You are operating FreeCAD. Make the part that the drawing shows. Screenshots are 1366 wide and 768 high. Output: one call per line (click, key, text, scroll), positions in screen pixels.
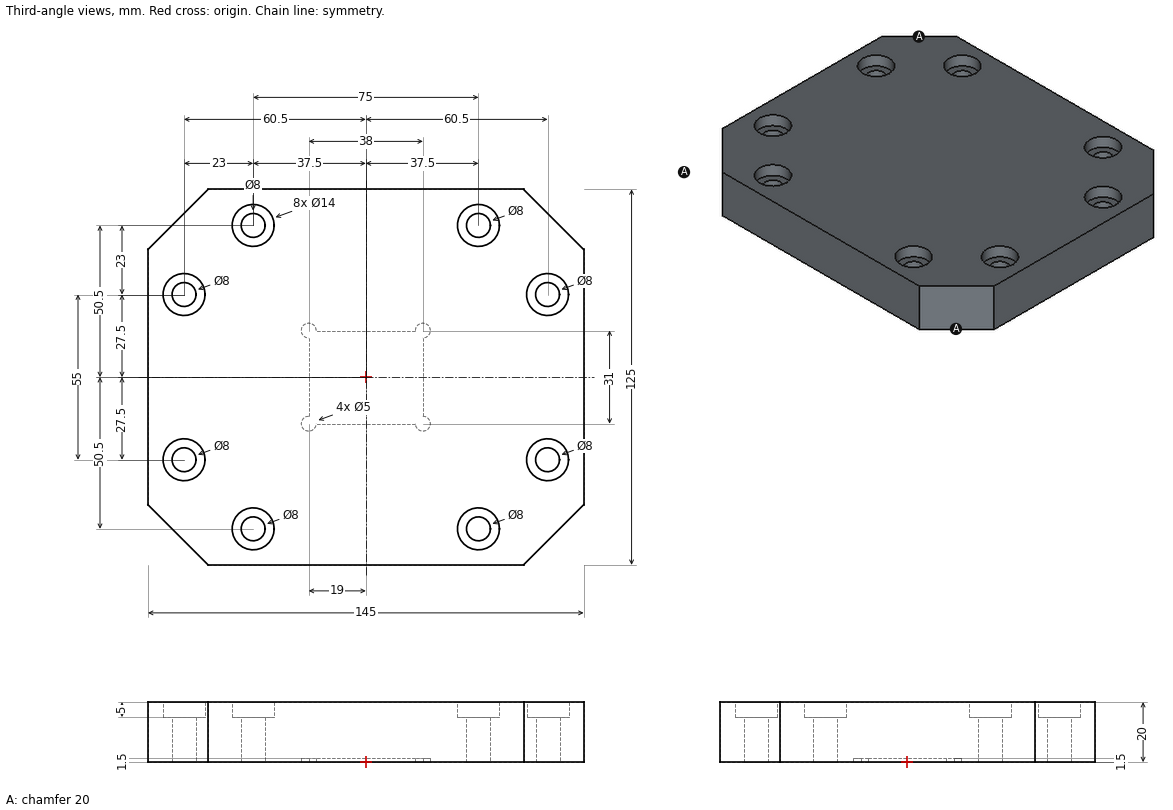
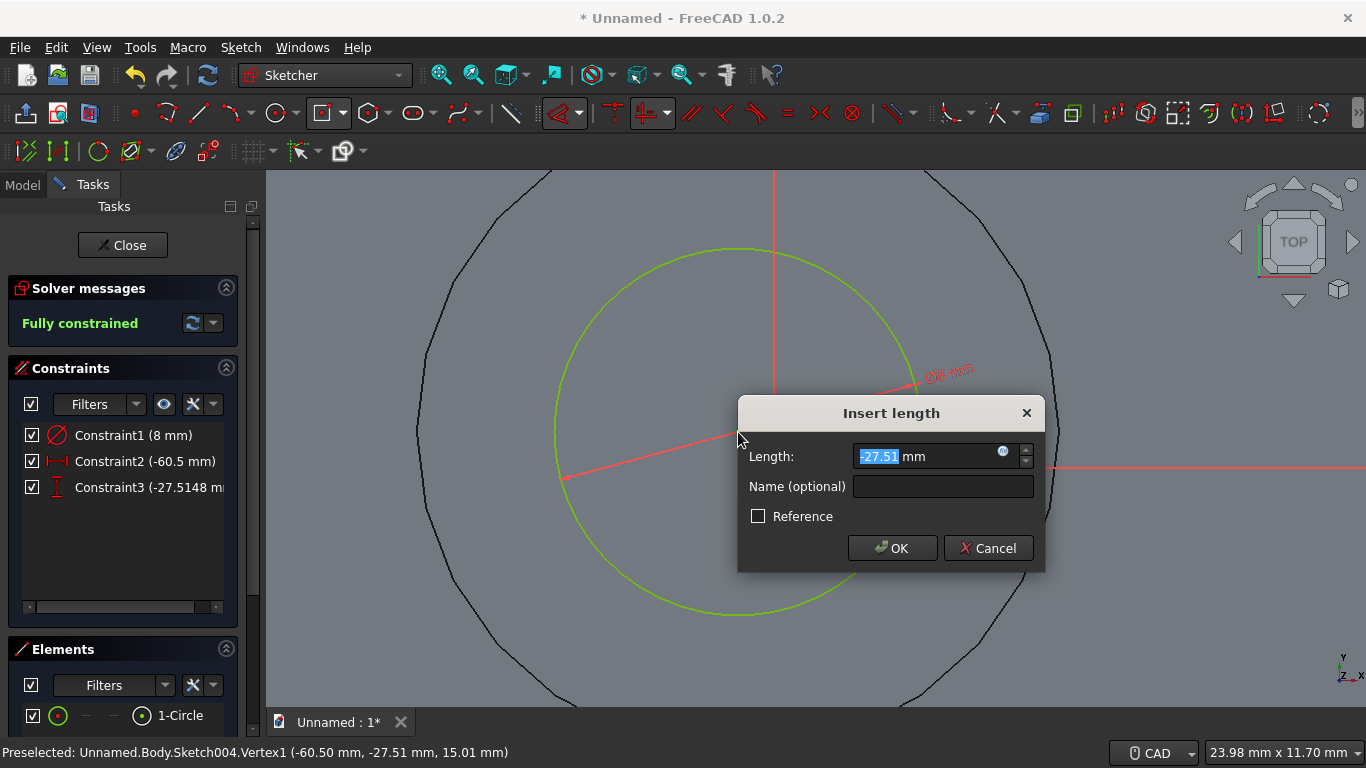
text(-27.5)
key(Return)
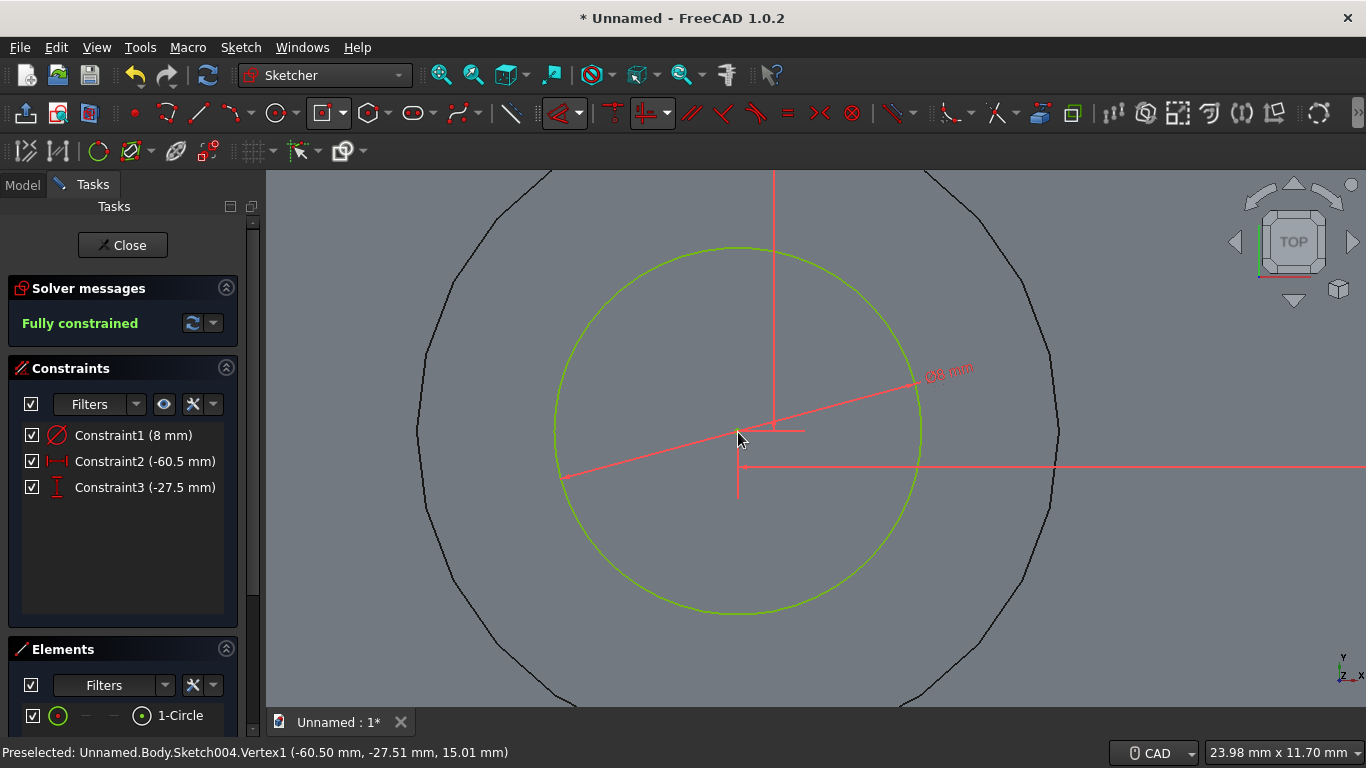
click(123, 245)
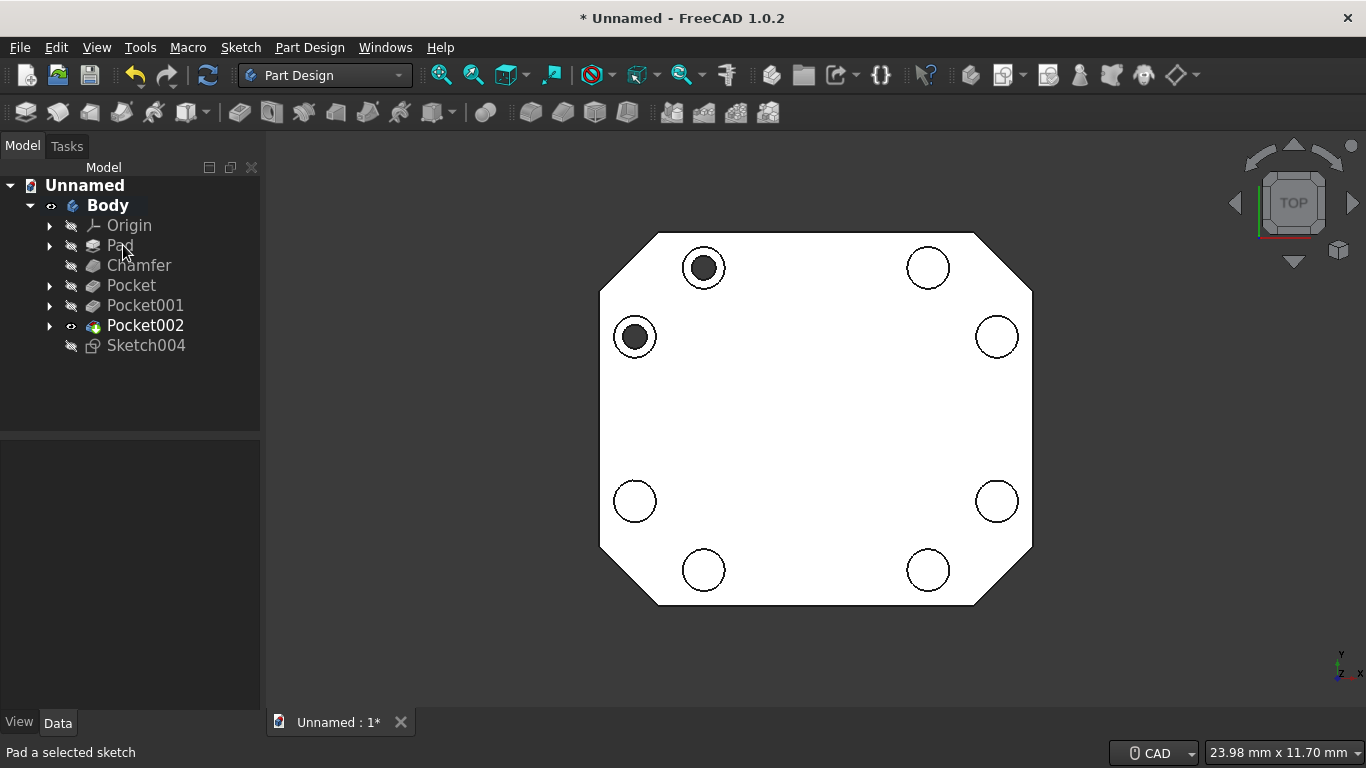
click(240, 112)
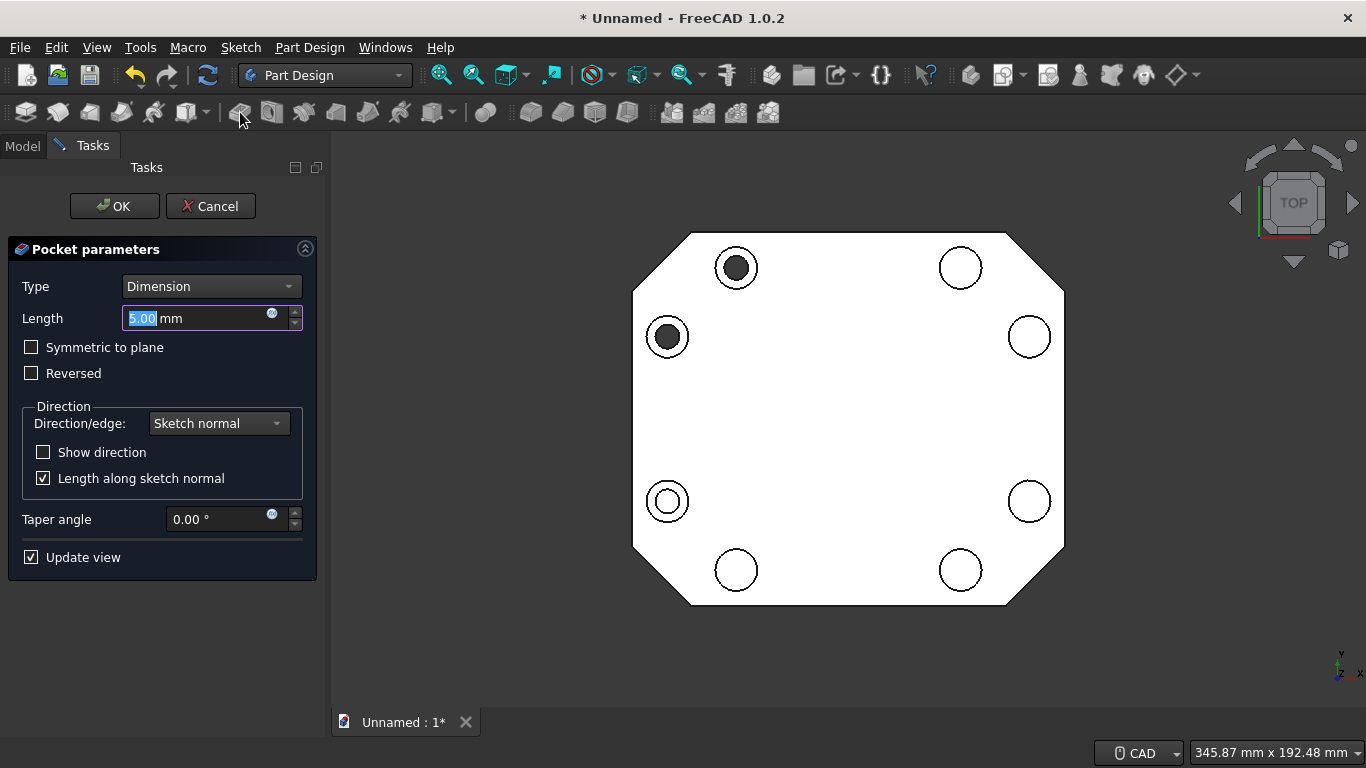
click(212, 286)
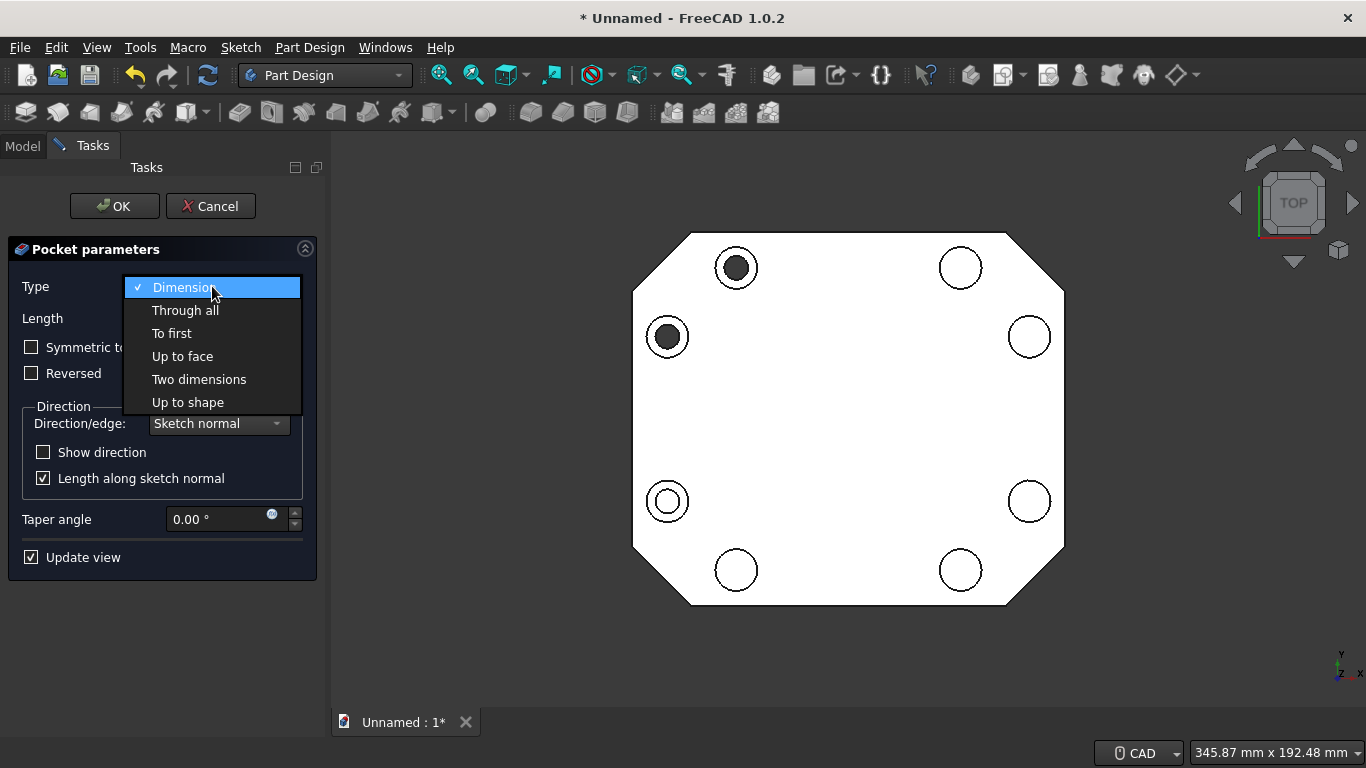
click(212, 334)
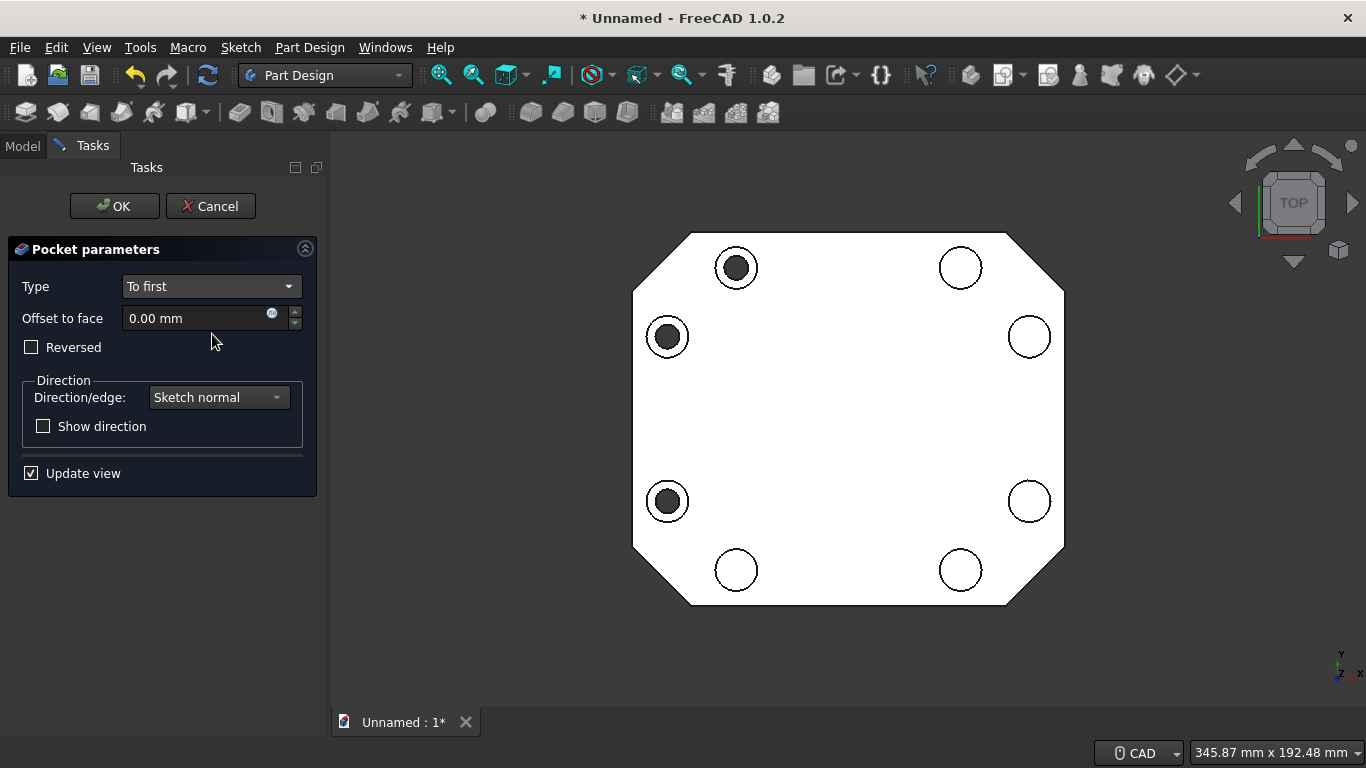
click(115, 206)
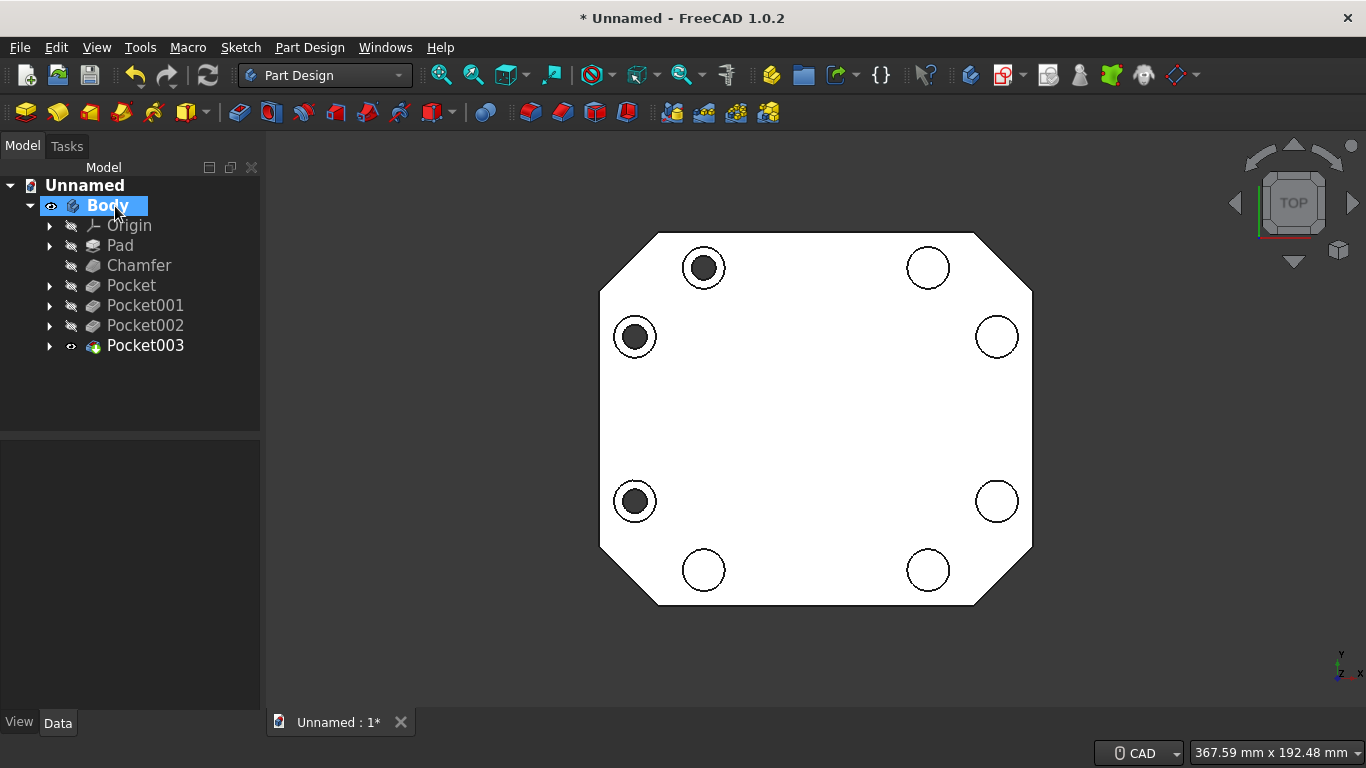
click(928, 267)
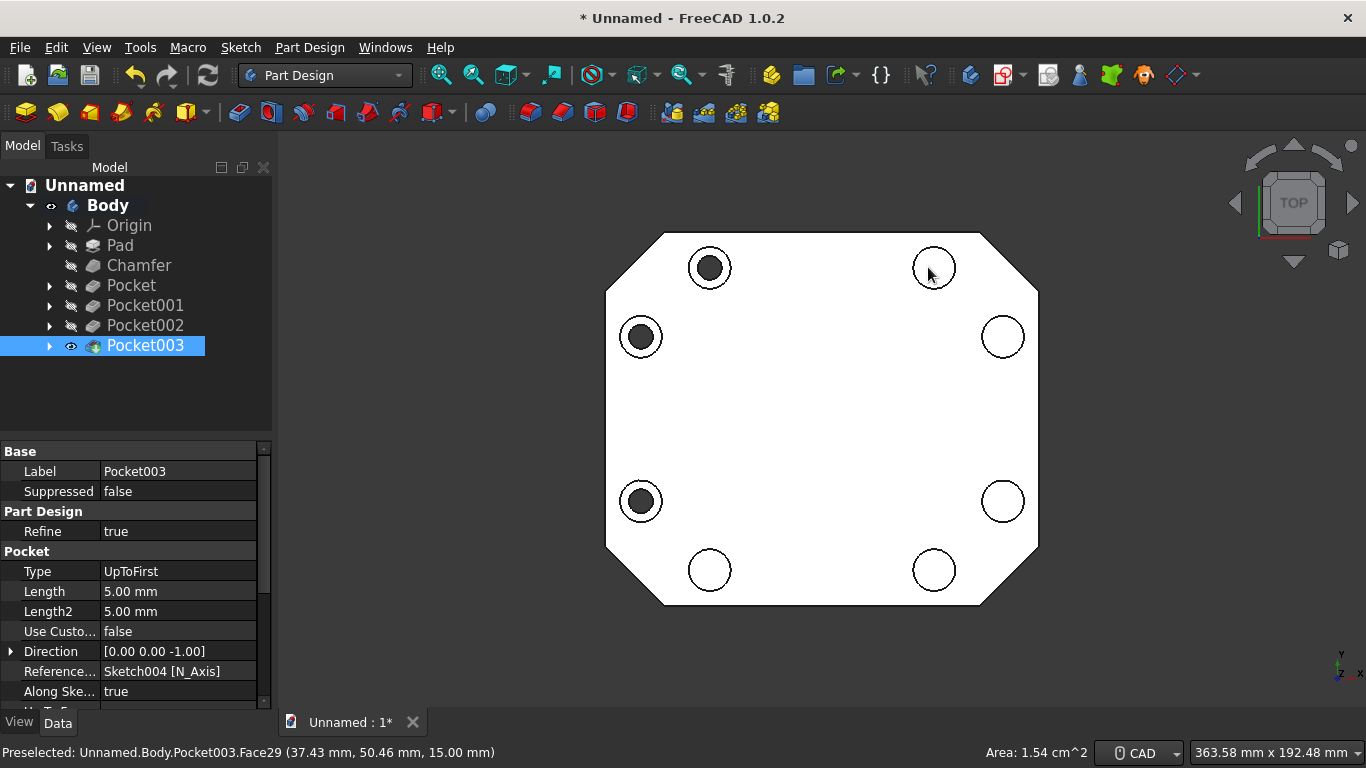
click(1004, 76)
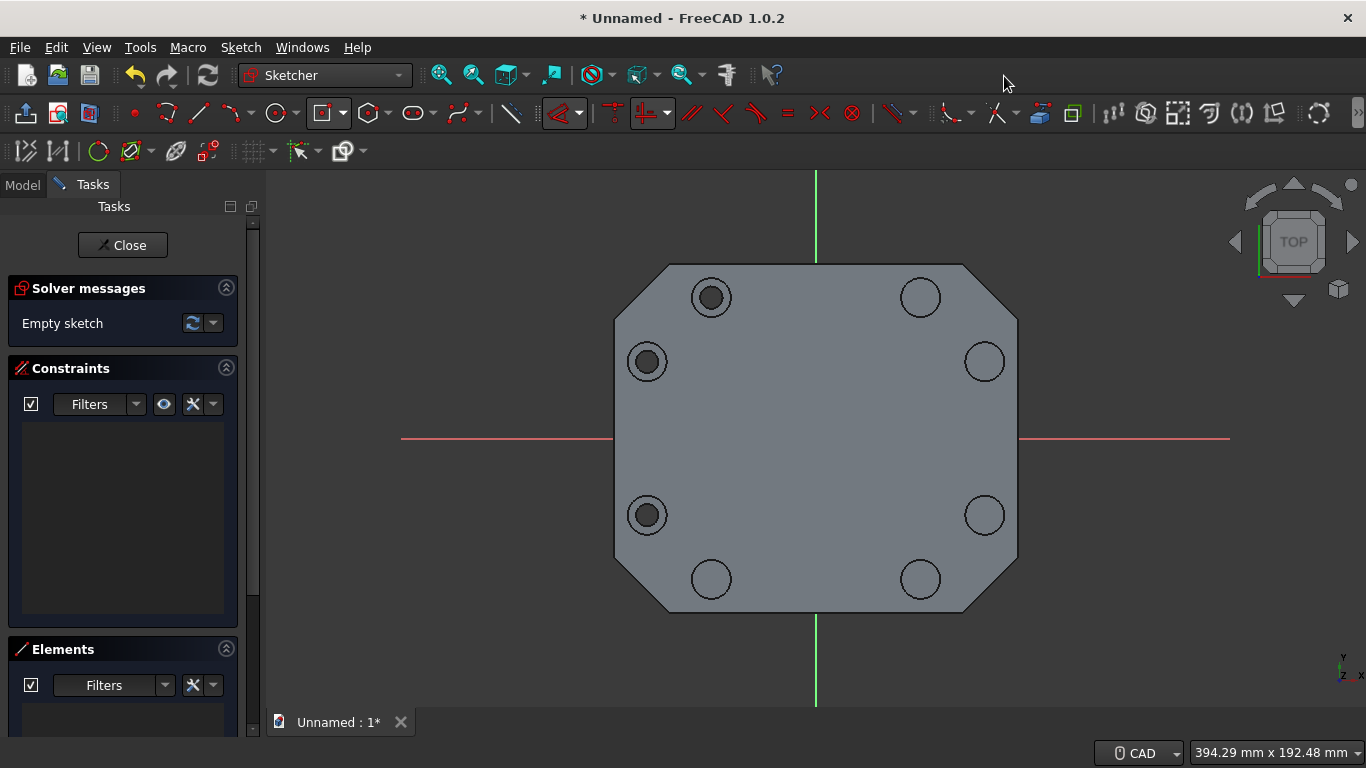
scroll(709, 589, up, 14)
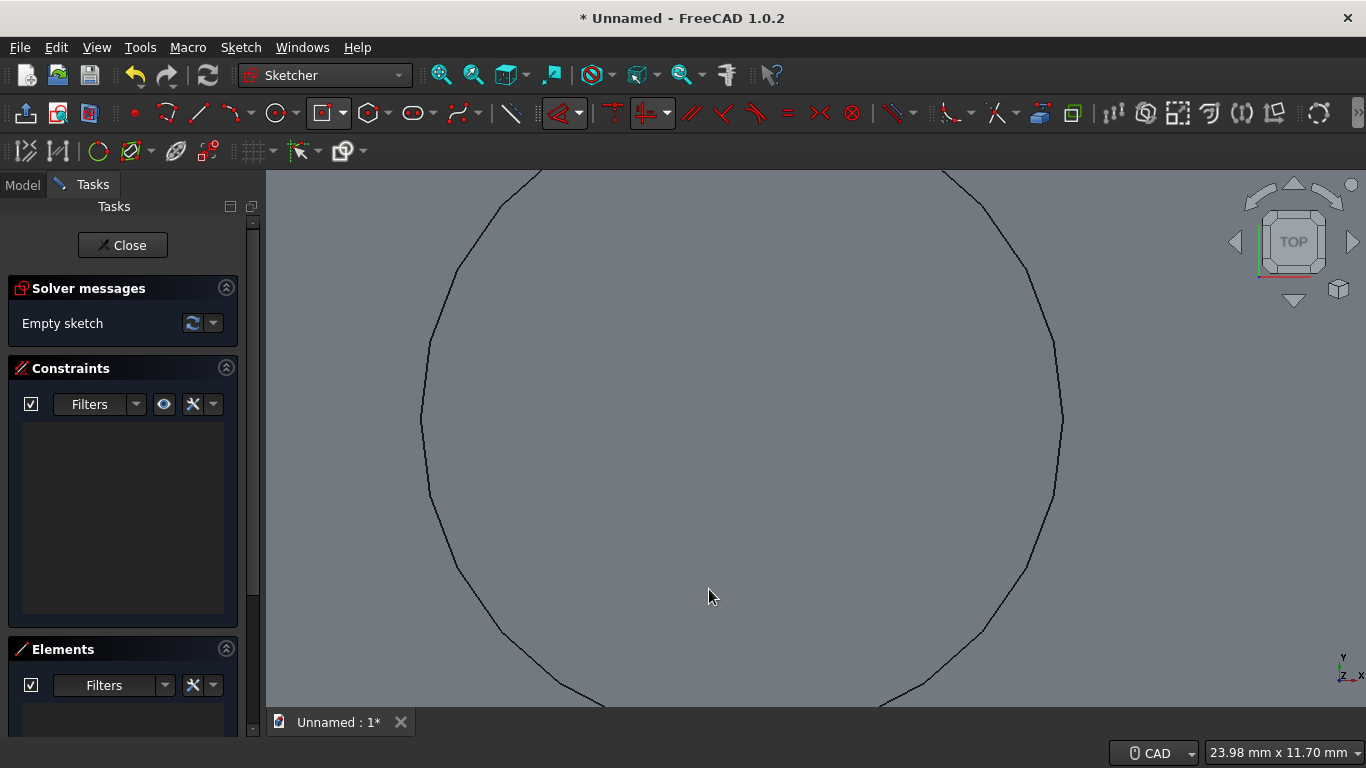
key(g)
key(c)